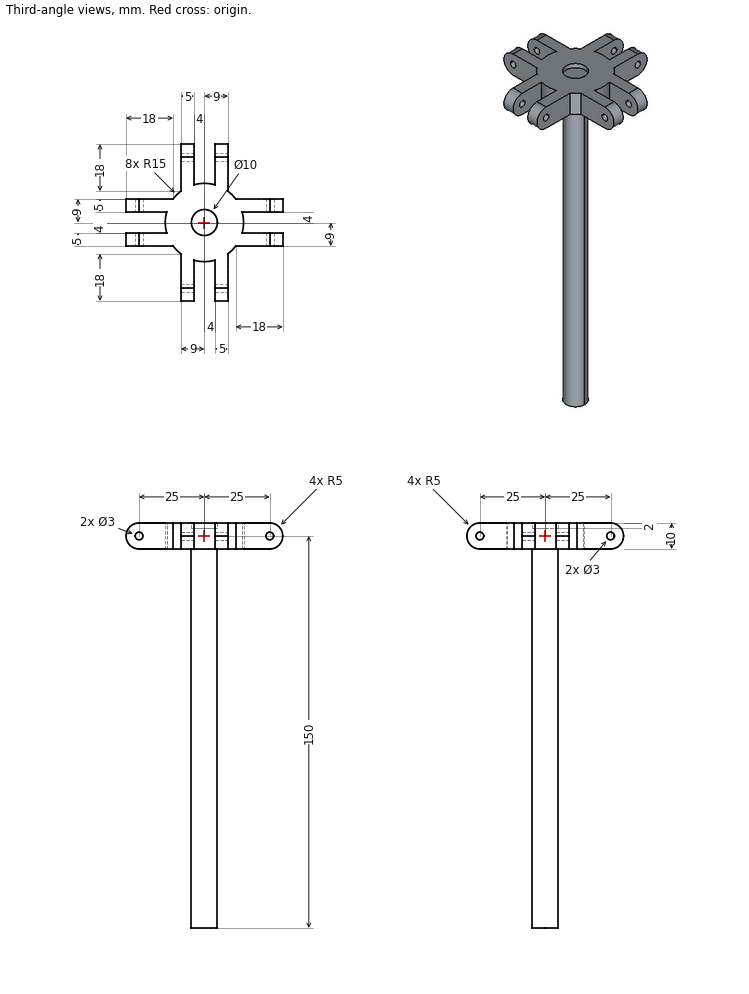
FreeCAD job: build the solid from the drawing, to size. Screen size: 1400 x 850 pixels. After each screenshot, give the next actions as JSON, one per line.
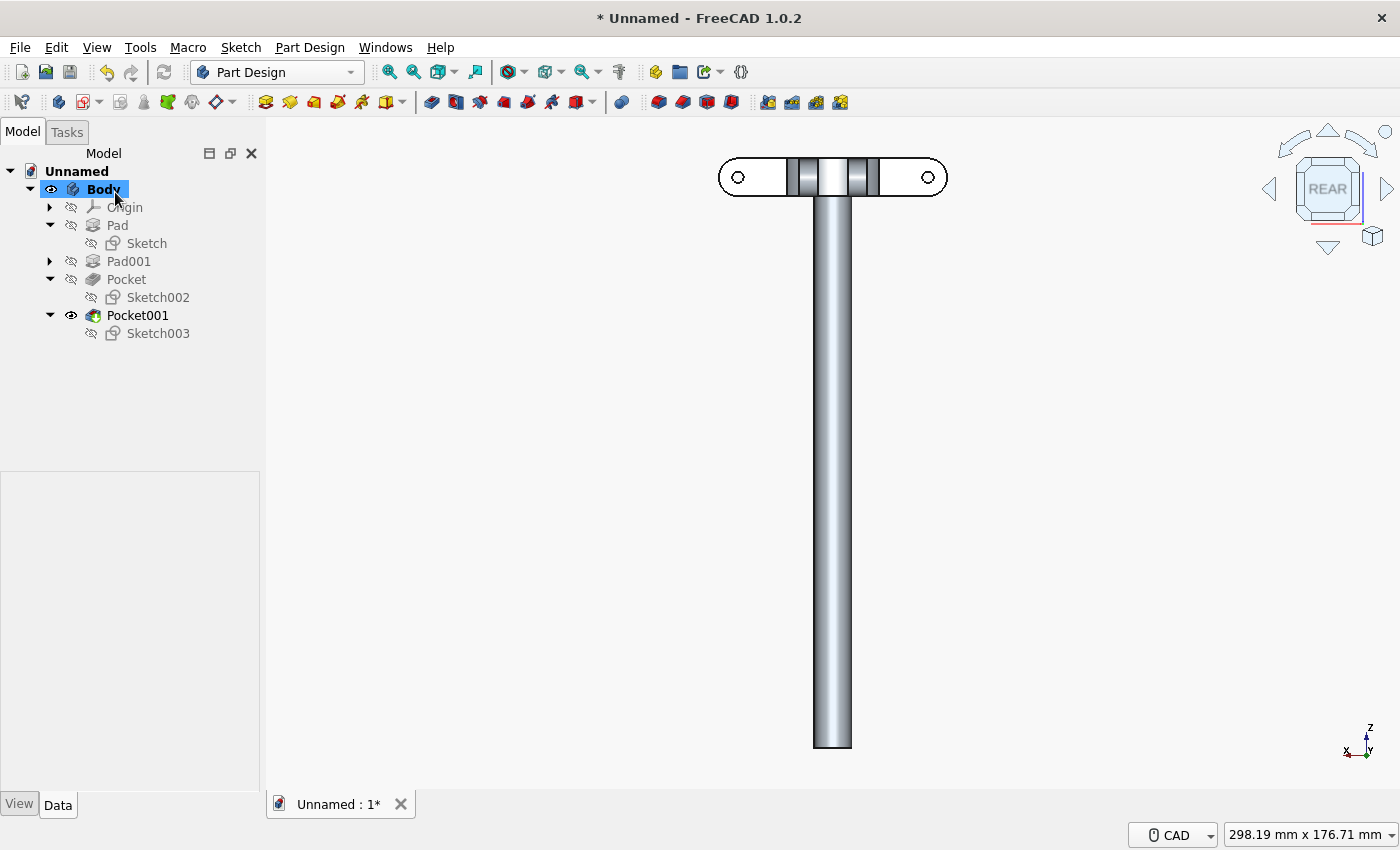
{"action": "key", "text": "0"}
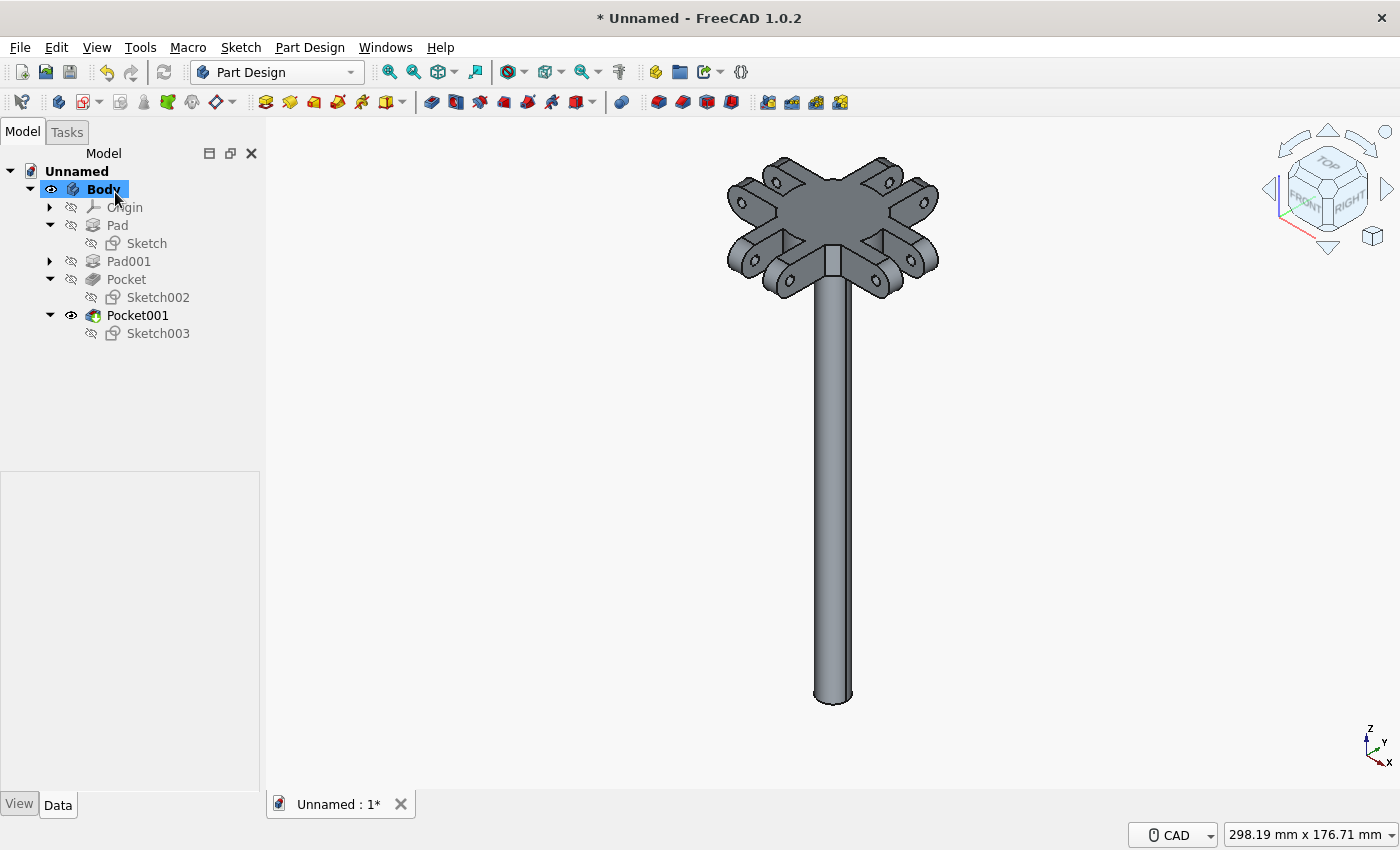
{"action": "left_click", "coordinate": [833, 211]}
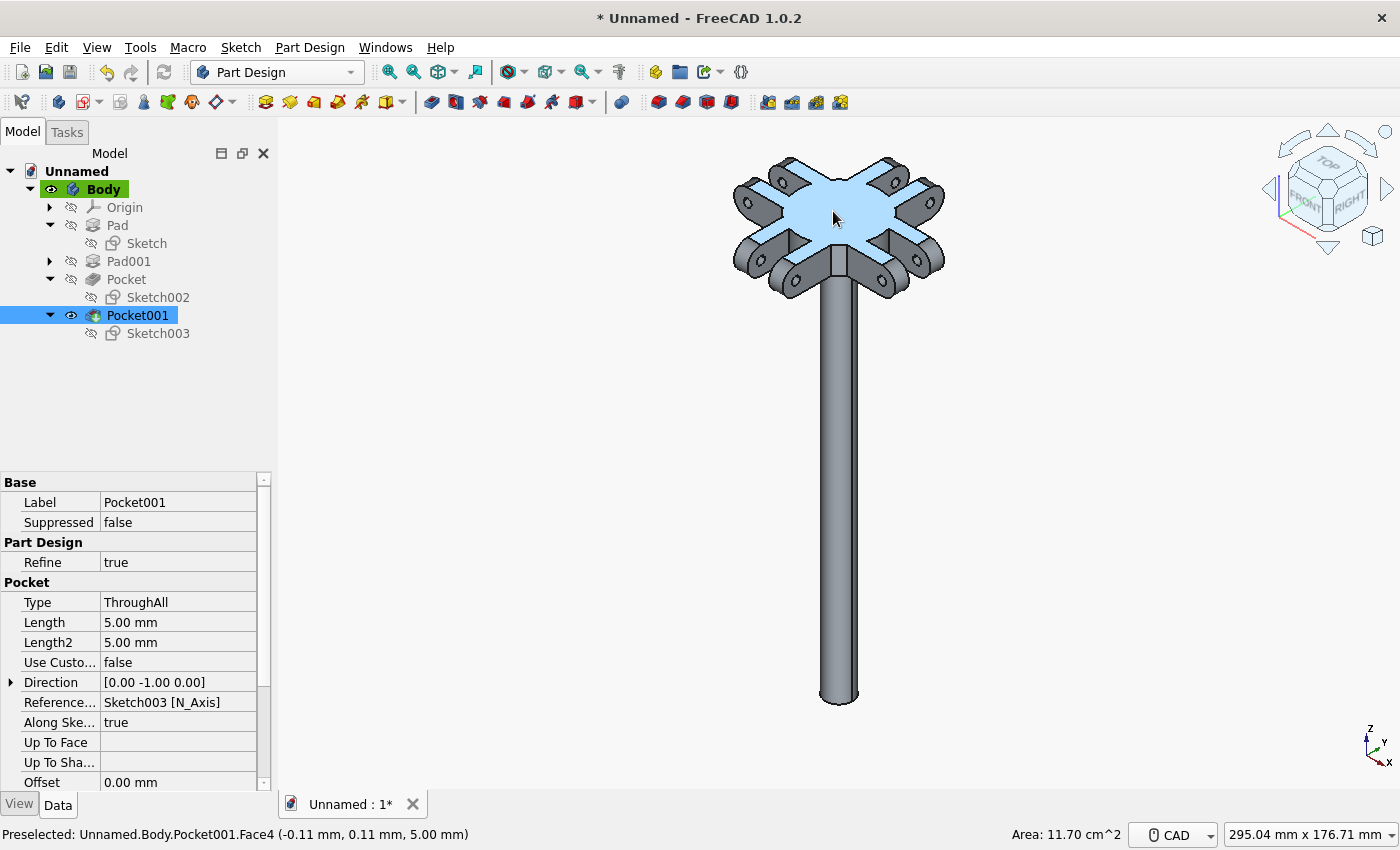
{"action": "left_click", "coordinate": [84, 102]}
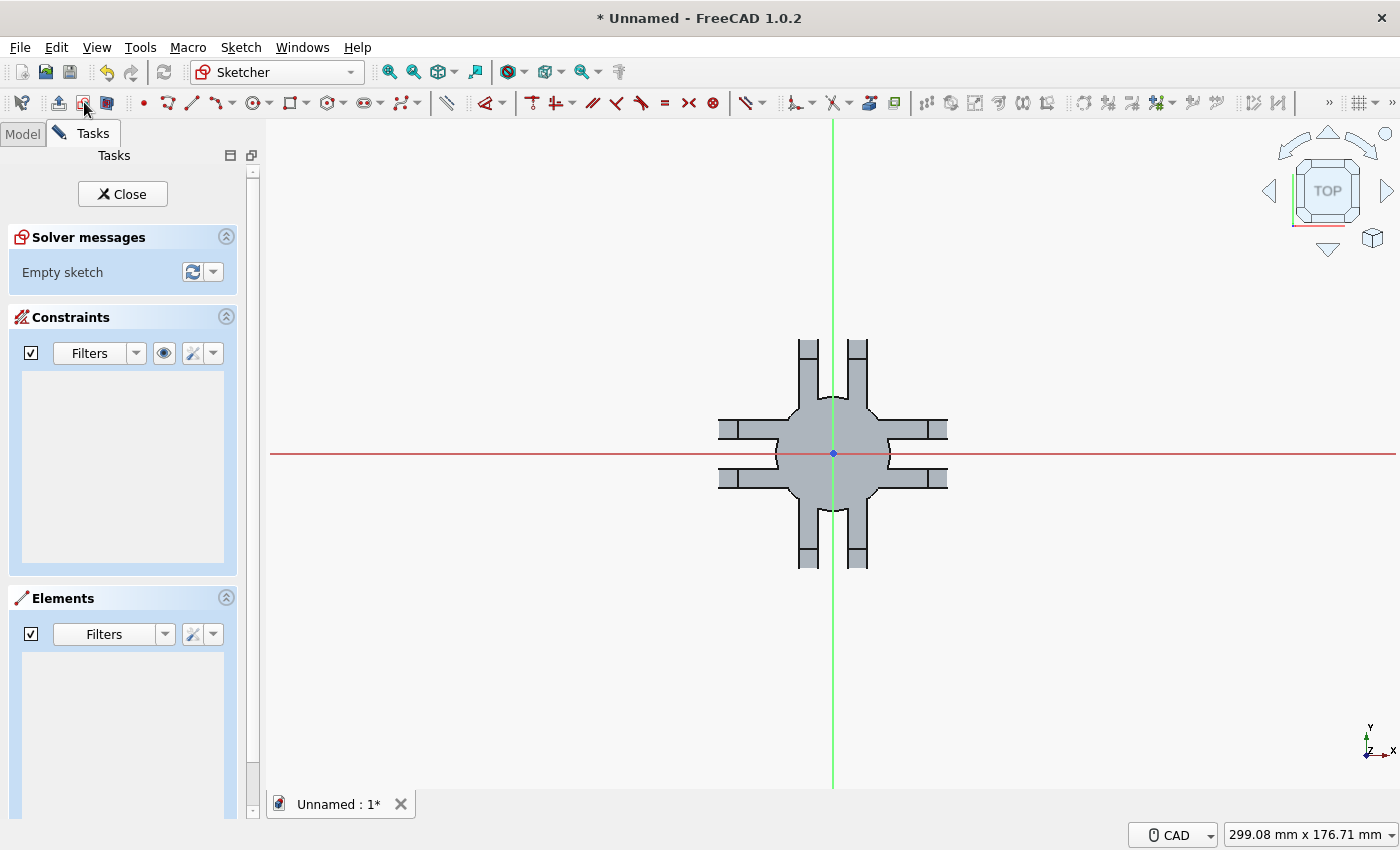
{"action": "scroll", "coordinate": [840, 454], "scroll_direction": "up", "scroll_amount": 12}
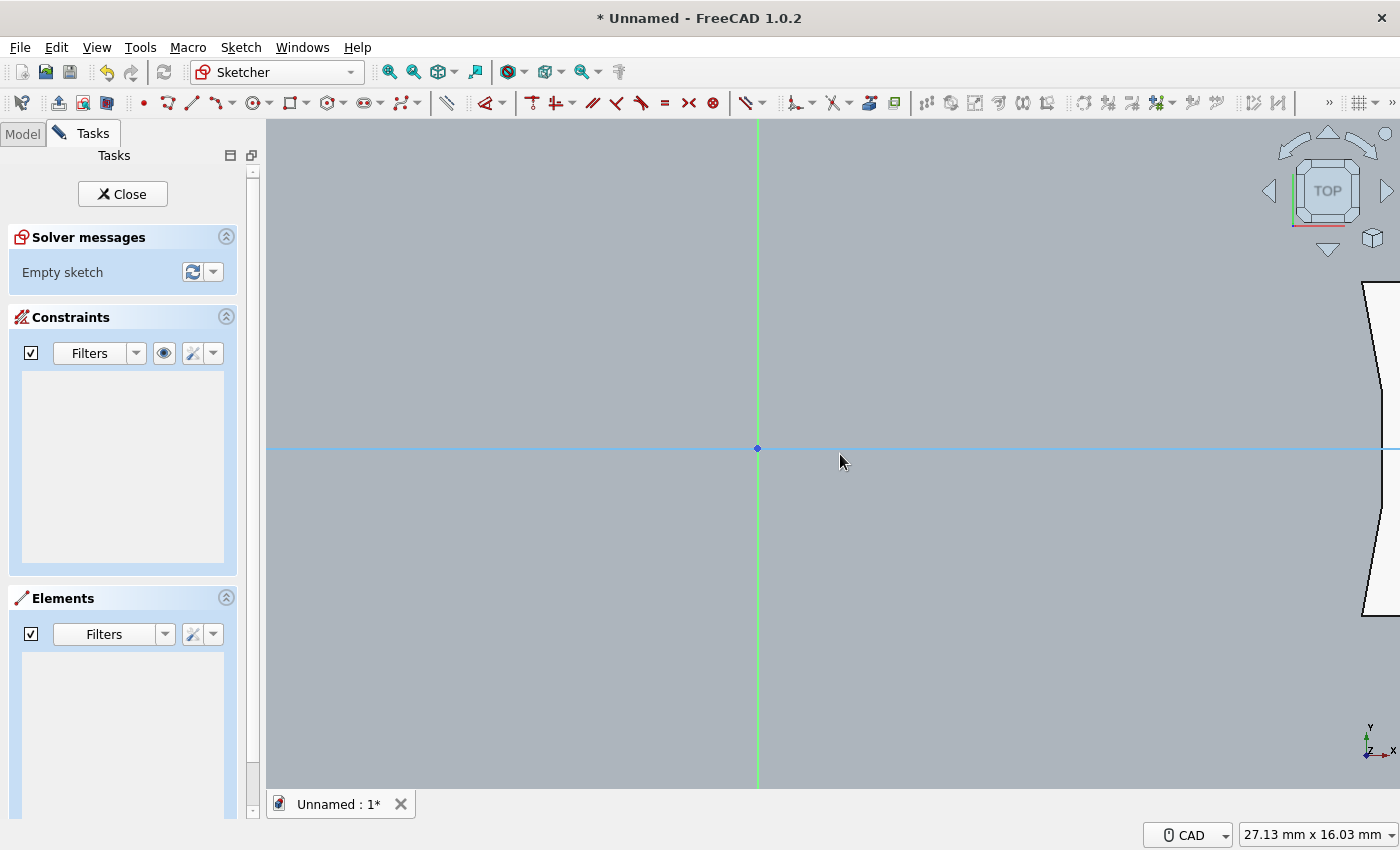
{"action": "left_click", "coordinate": [254, 104]}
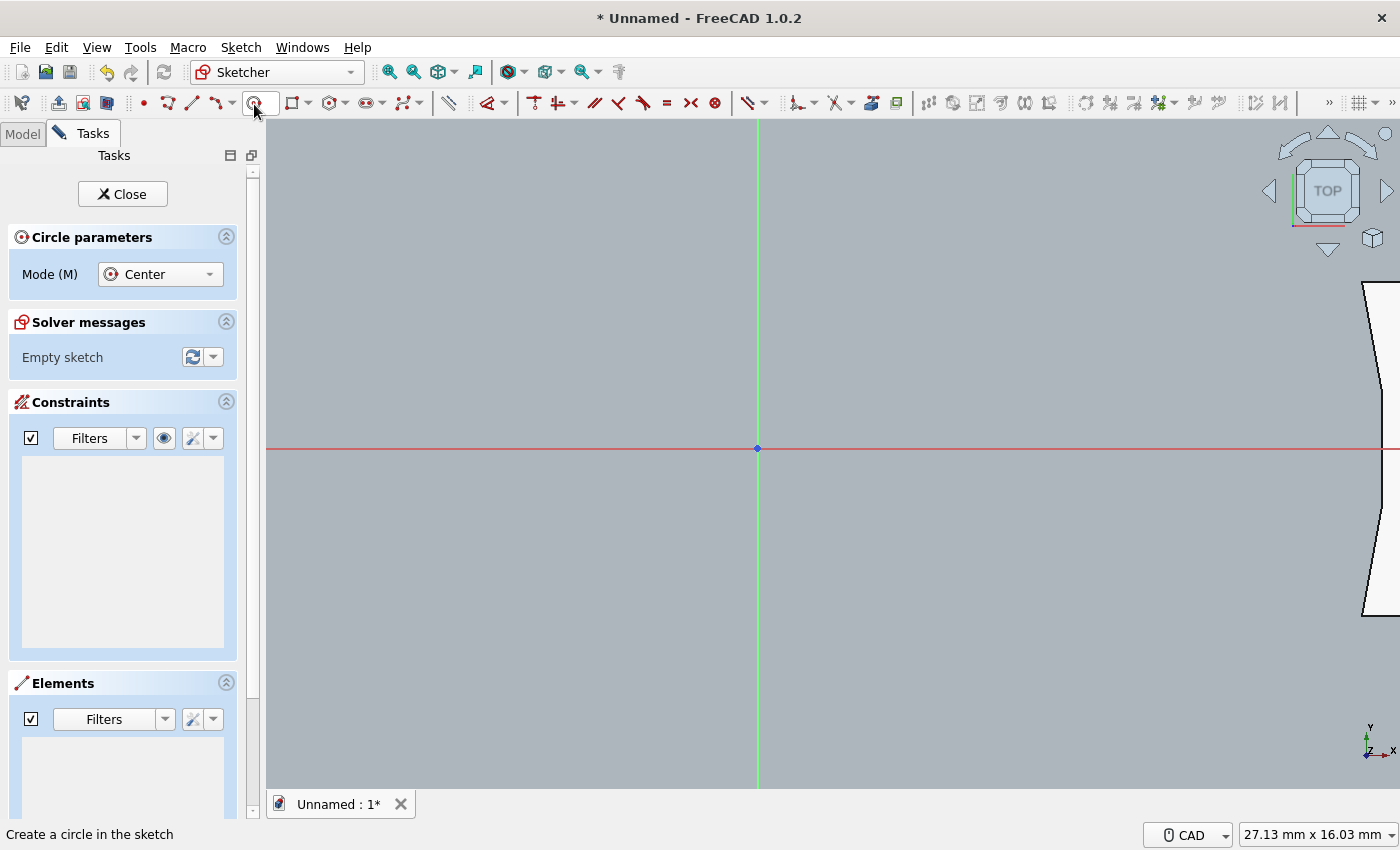
{"action": "left_click", "coordinate": [758, 449]}
{"action": "mouse_move", "coordinate": [906, 301]}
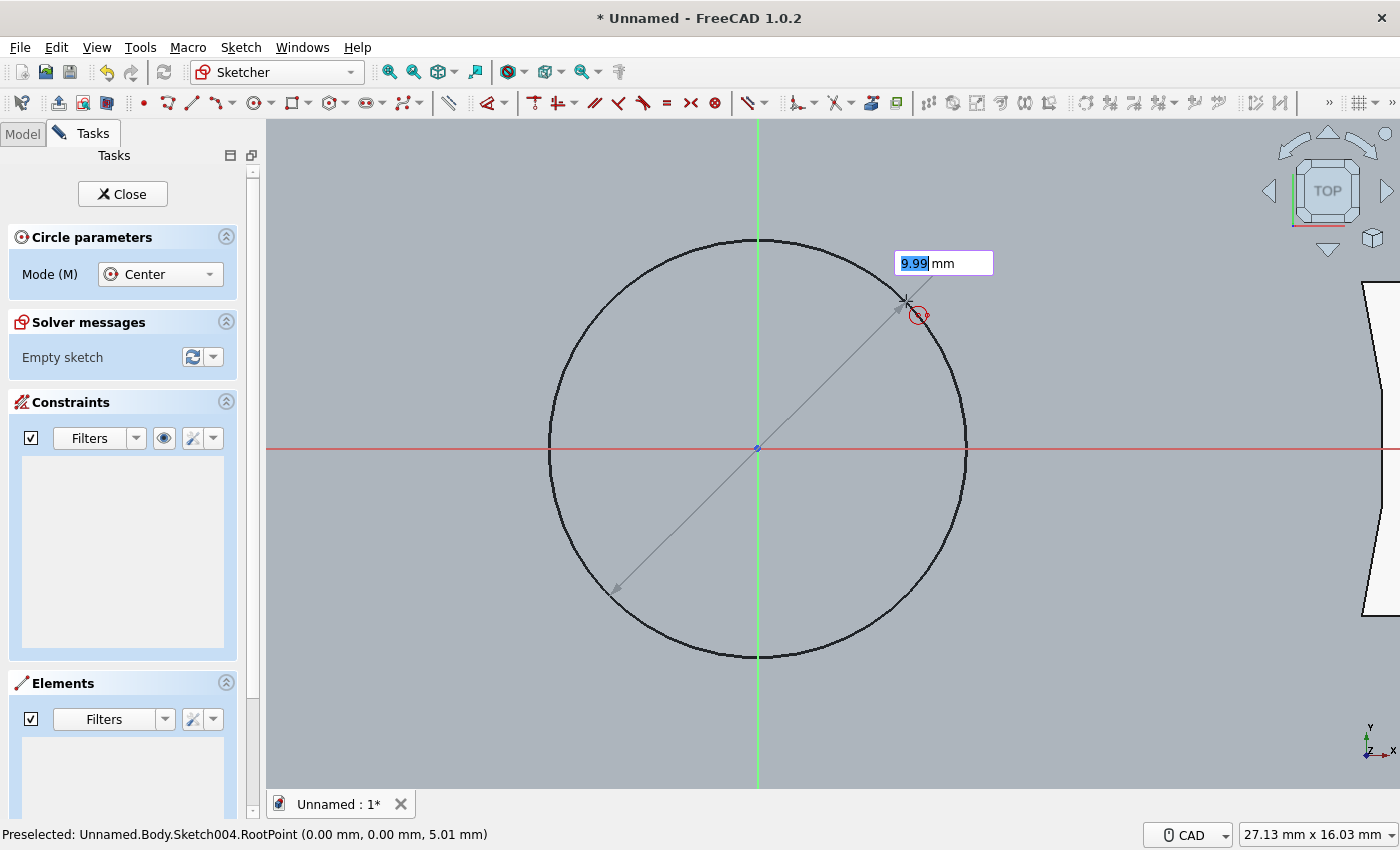
{"action": "type", "text": "10"}
{"action": "key", "text": "Return"}
{"action": "key", "text": "Escape"}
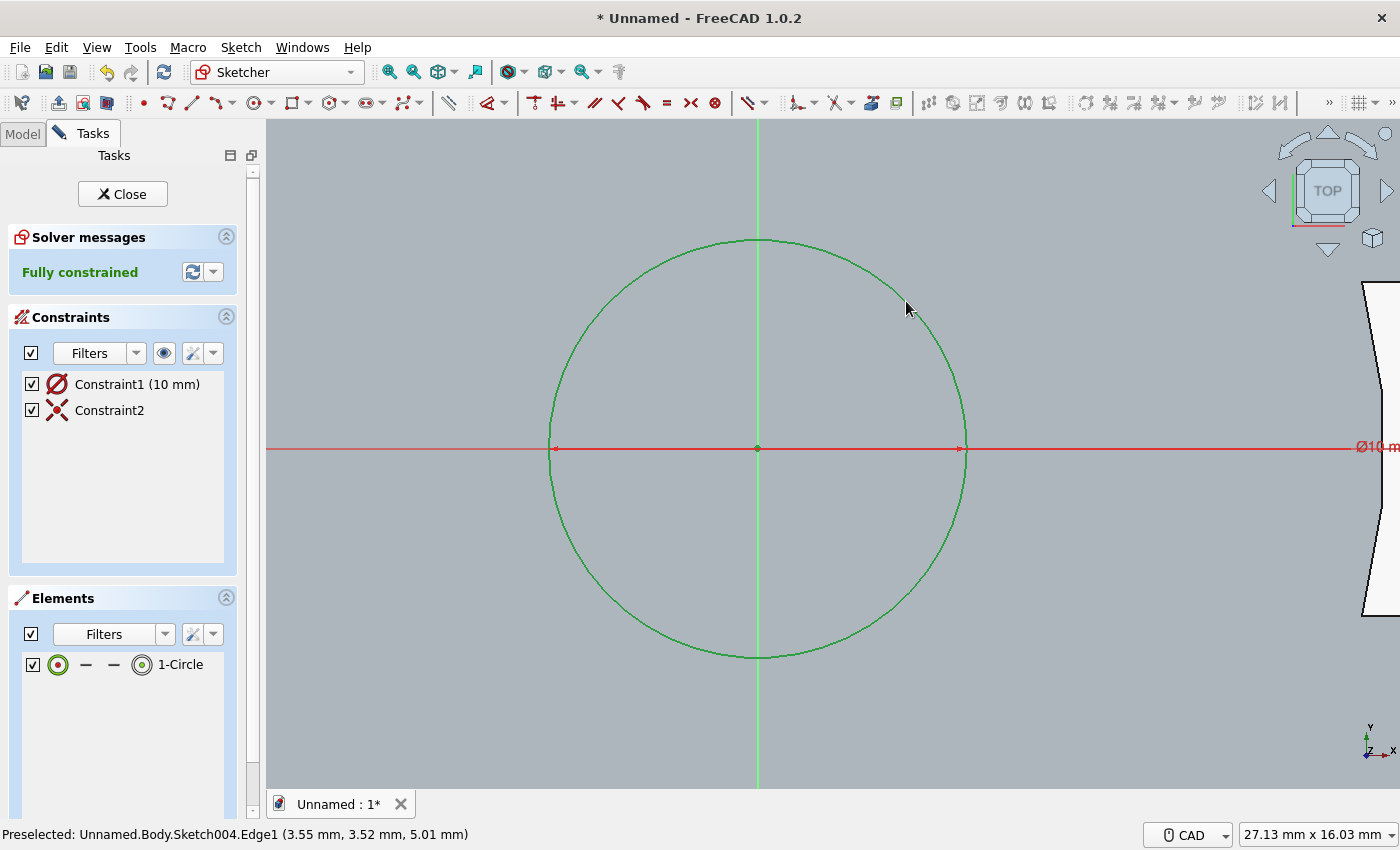
{"action": "left_click", "coordinate": [123, 194]}